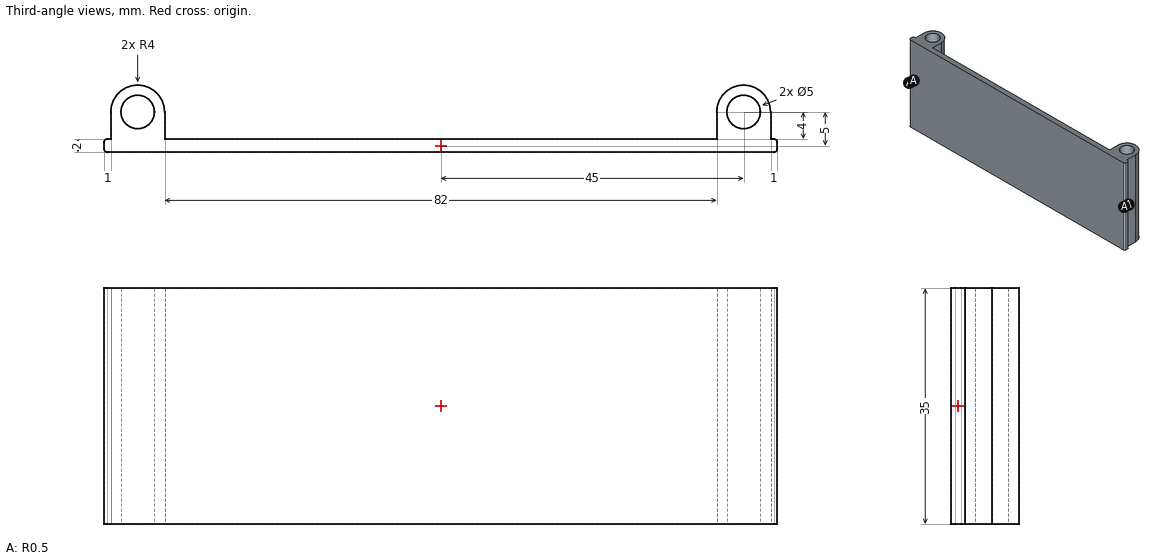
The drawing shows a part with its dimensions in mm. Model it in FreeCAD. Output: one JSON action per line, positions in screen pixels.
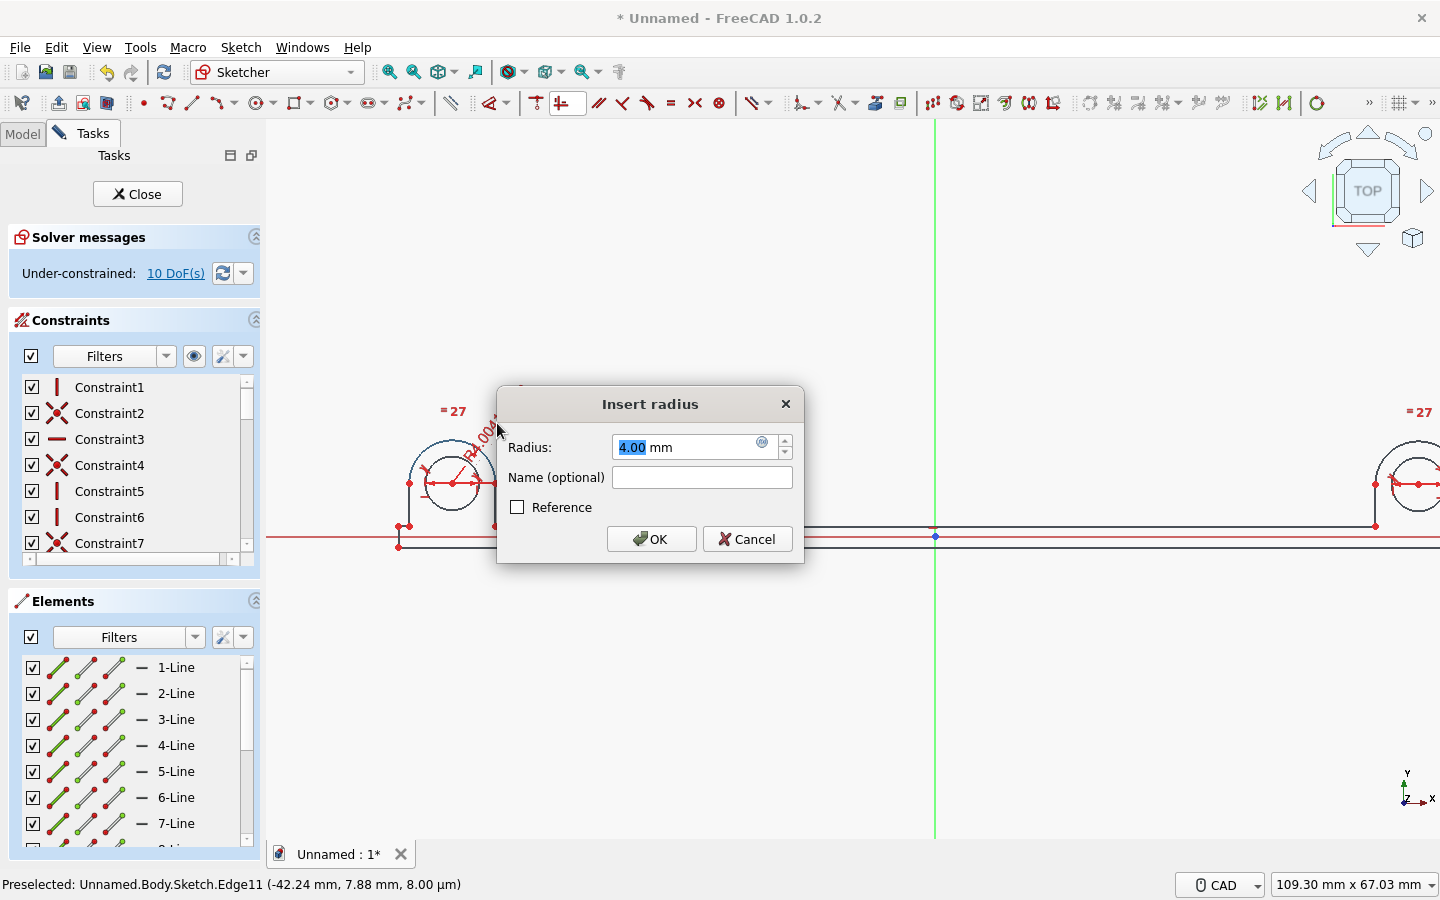
{"action": "type", "text": "4"}
{"action": "key", "text": "Return"}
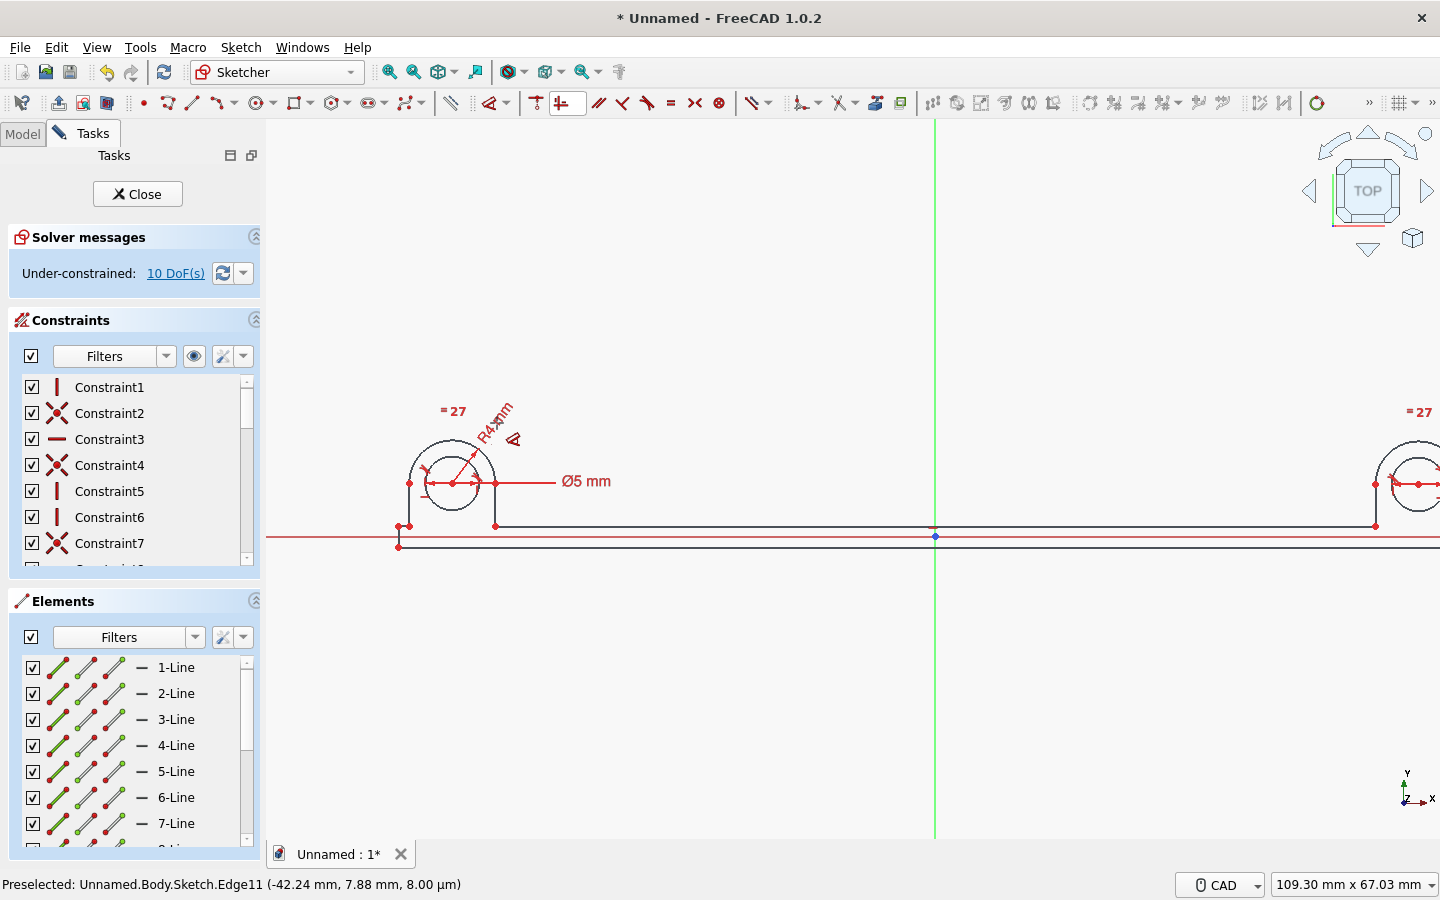
{"action": "scroll", "coordinate": [478, 449], "scroll_direction": "down", "scroll_amount": 2}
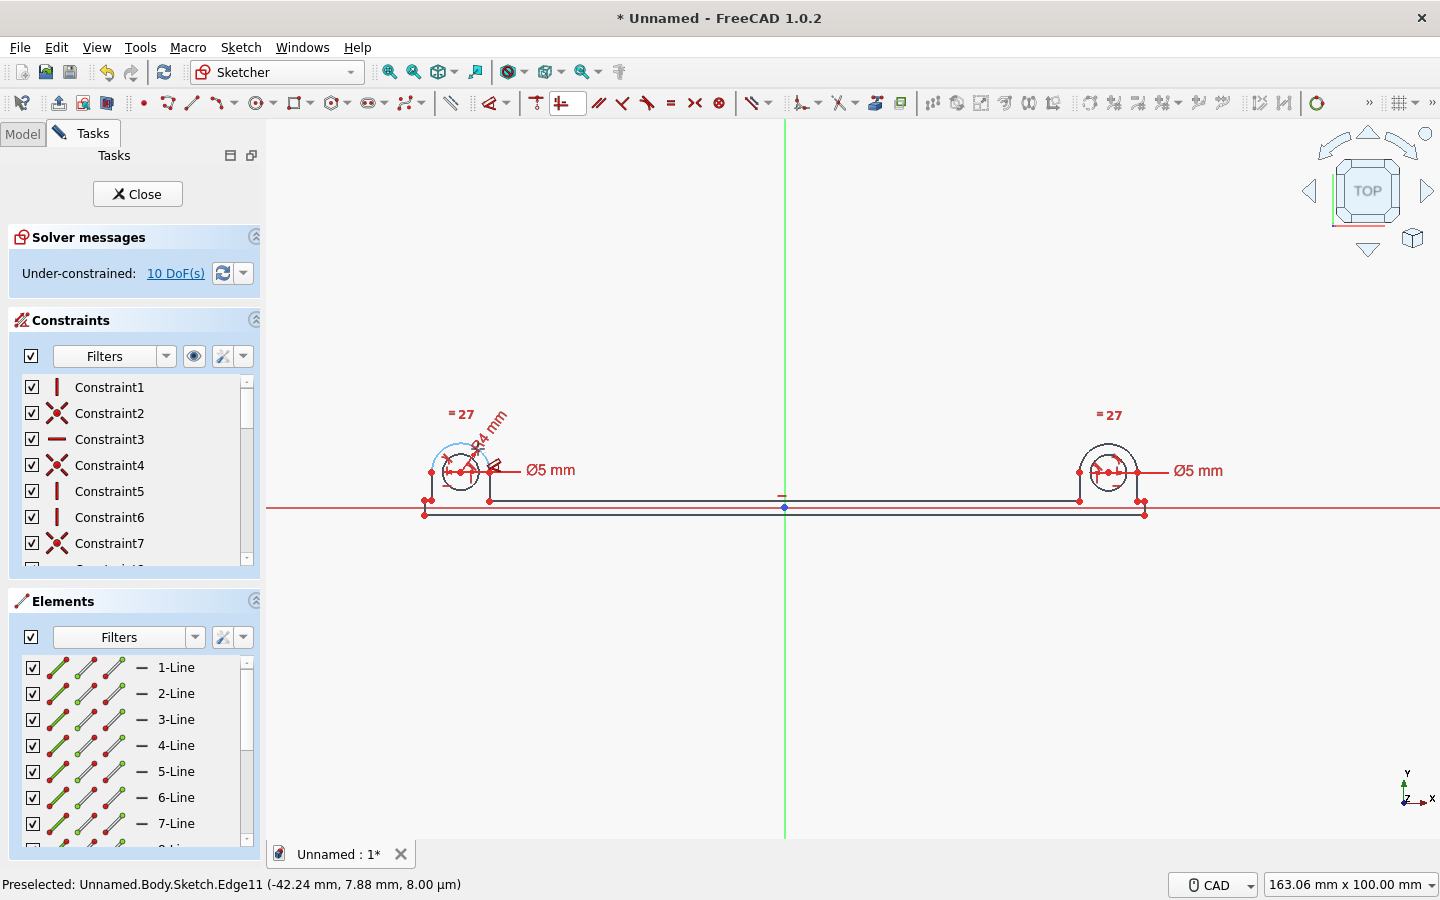
{"action": "scroll", "coordinate": [1080, 481], "scroll_direction": "up", "scroll_amount": 3}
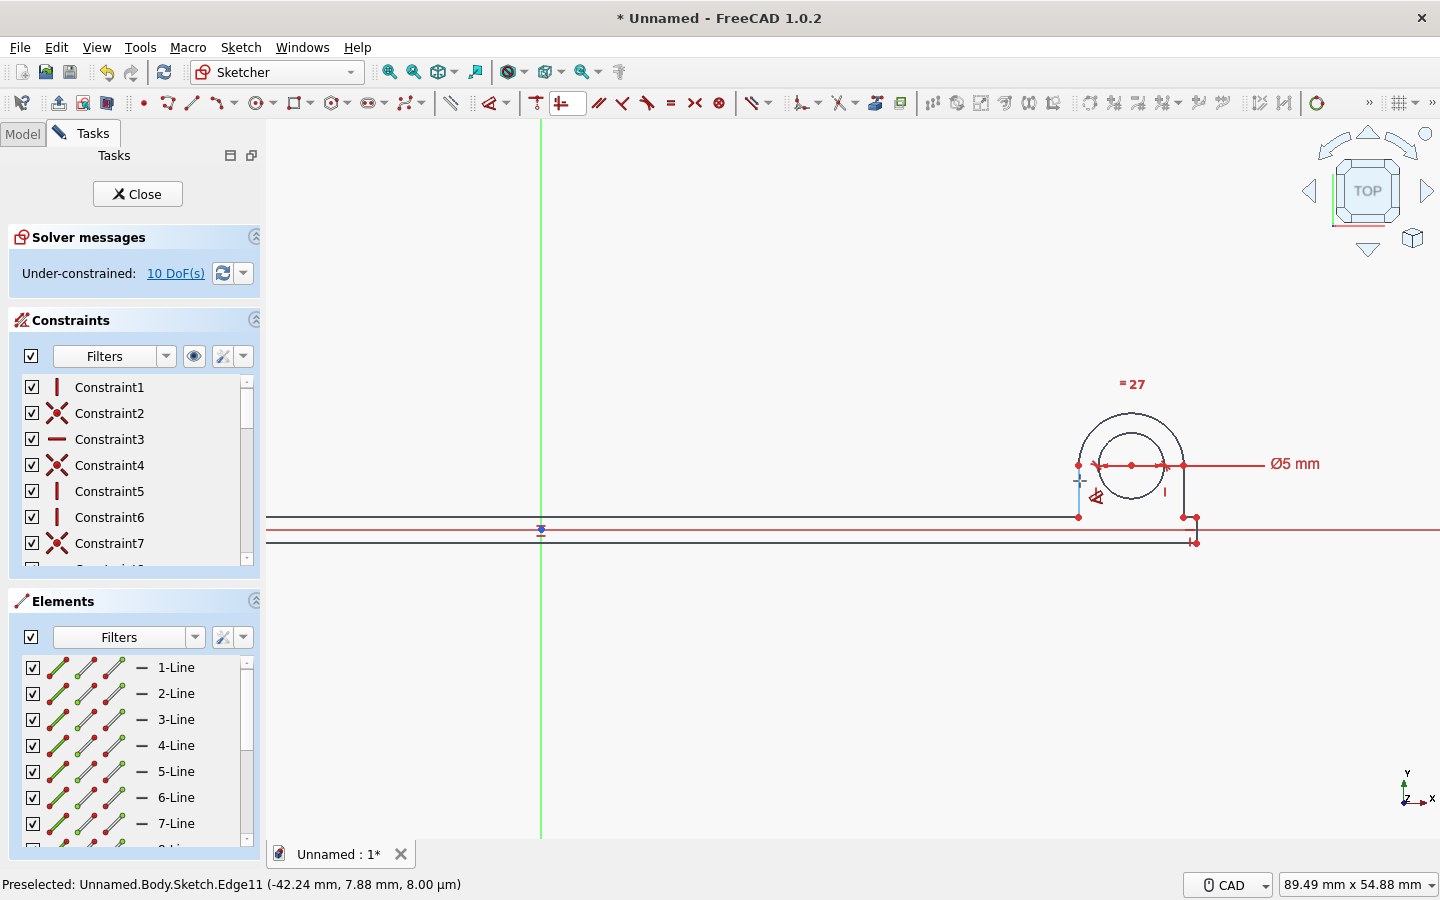
{"action": "left_click", "coordinate": [1079, 481]}
{"action": "left_click", "coordinate": [1113, 510]}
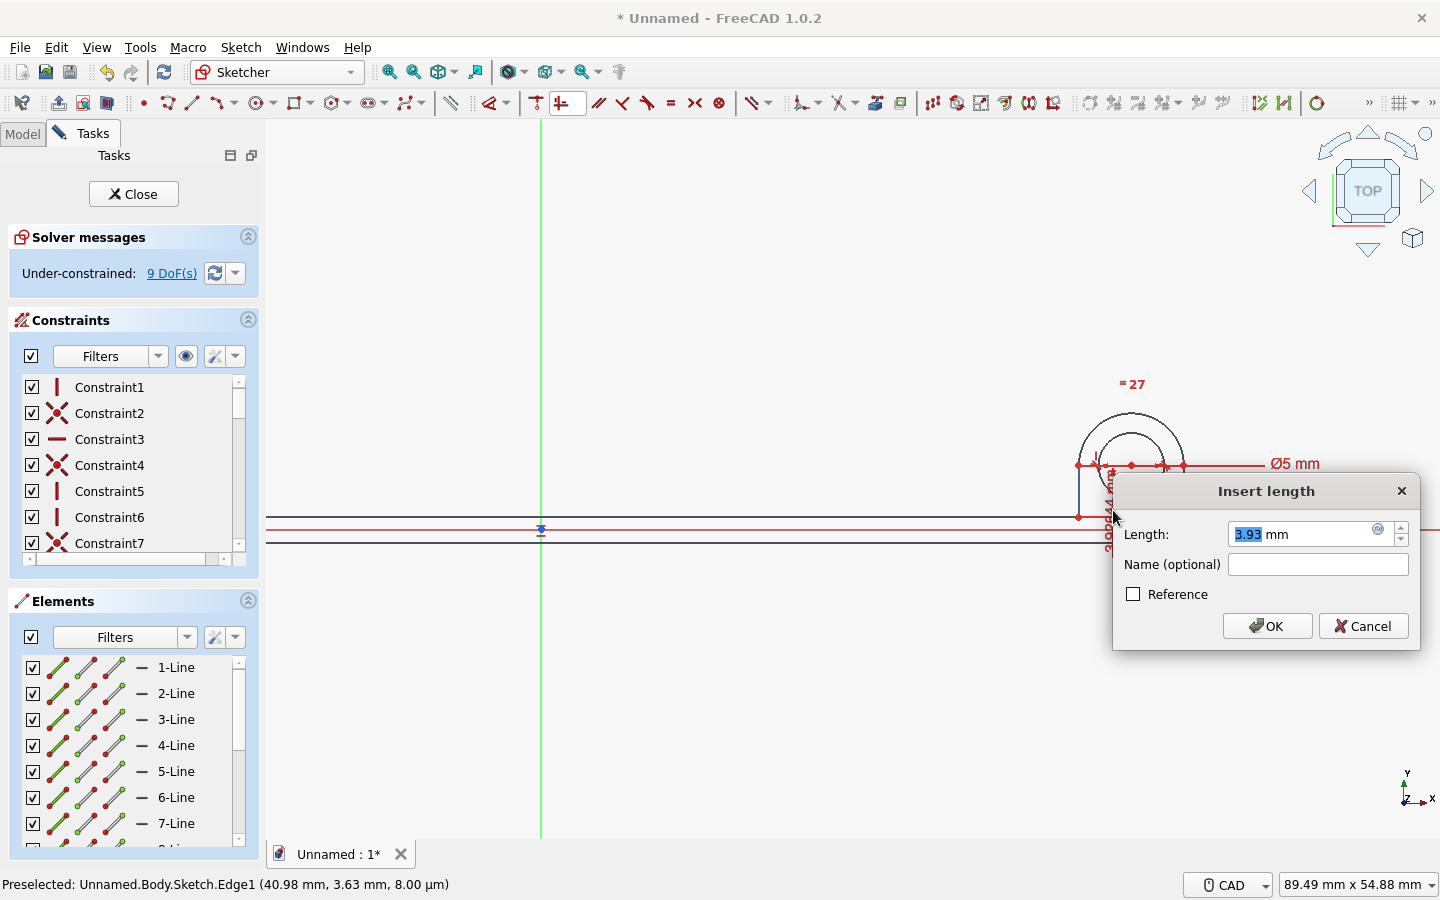
{"action": "type", "text": "4"}
{"action": "key", "text": "Return"}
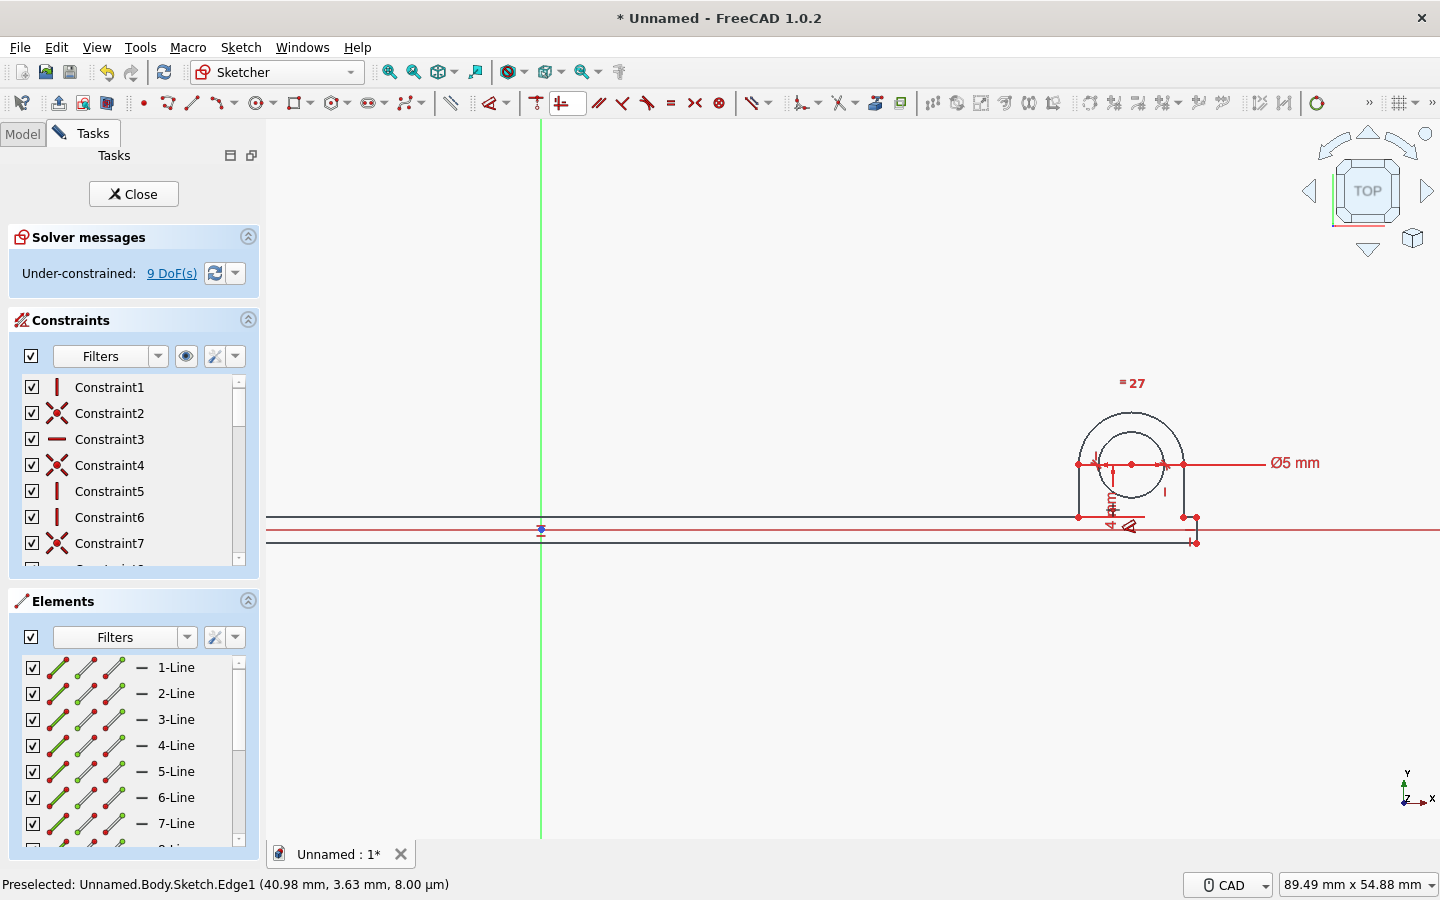
{"action": "scroll", "coordinate": [1080, 481], "scroll_direction": "down", "scroll_amount": 3}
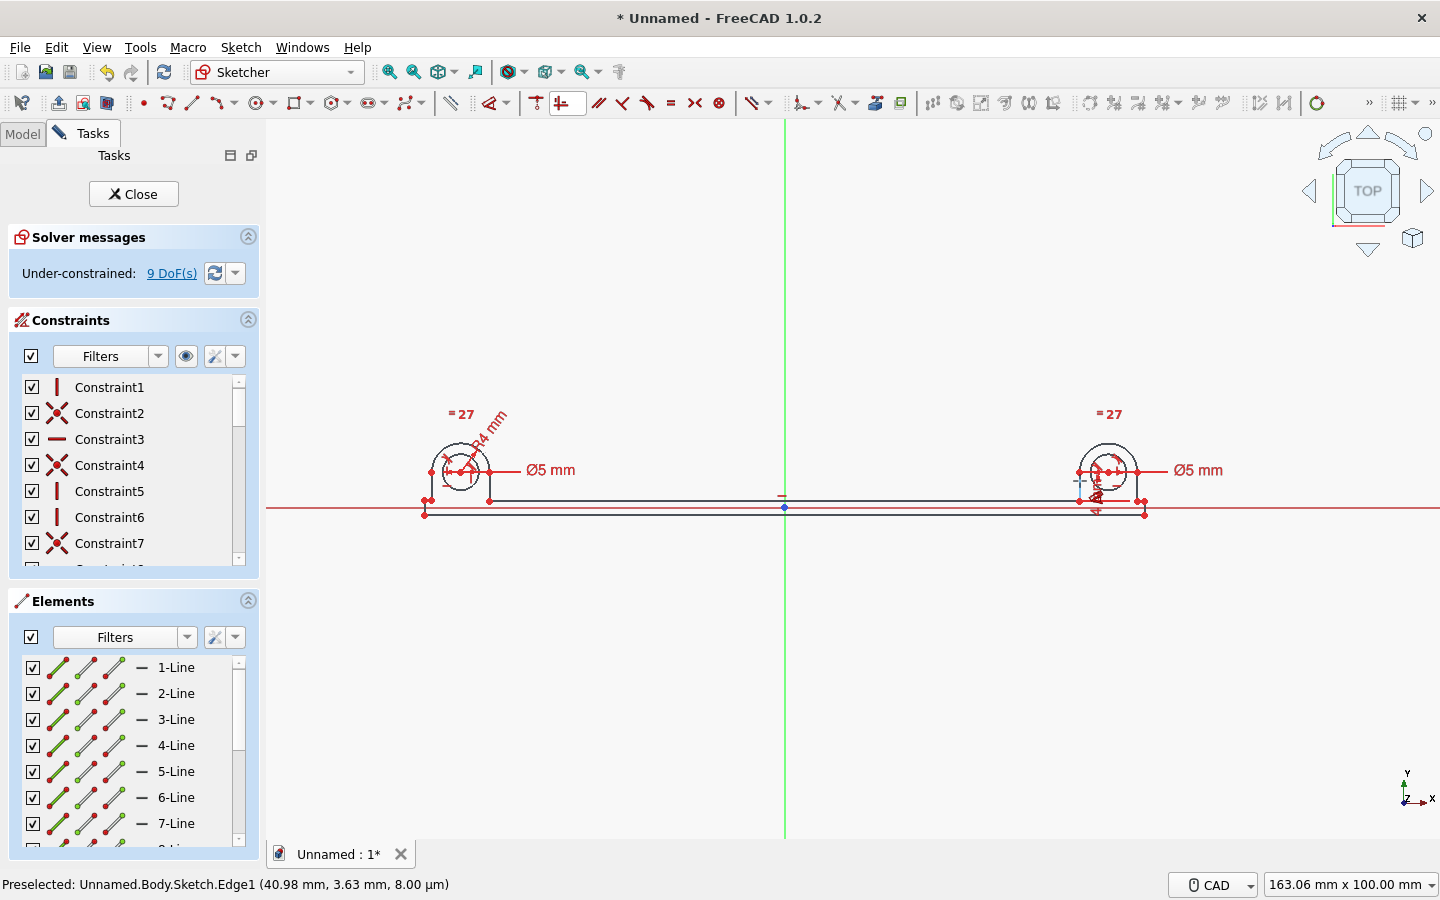
{"action": "scroll", "coordinate": [490, 493], "scroll_direction": "up", "scroll_amount": 3}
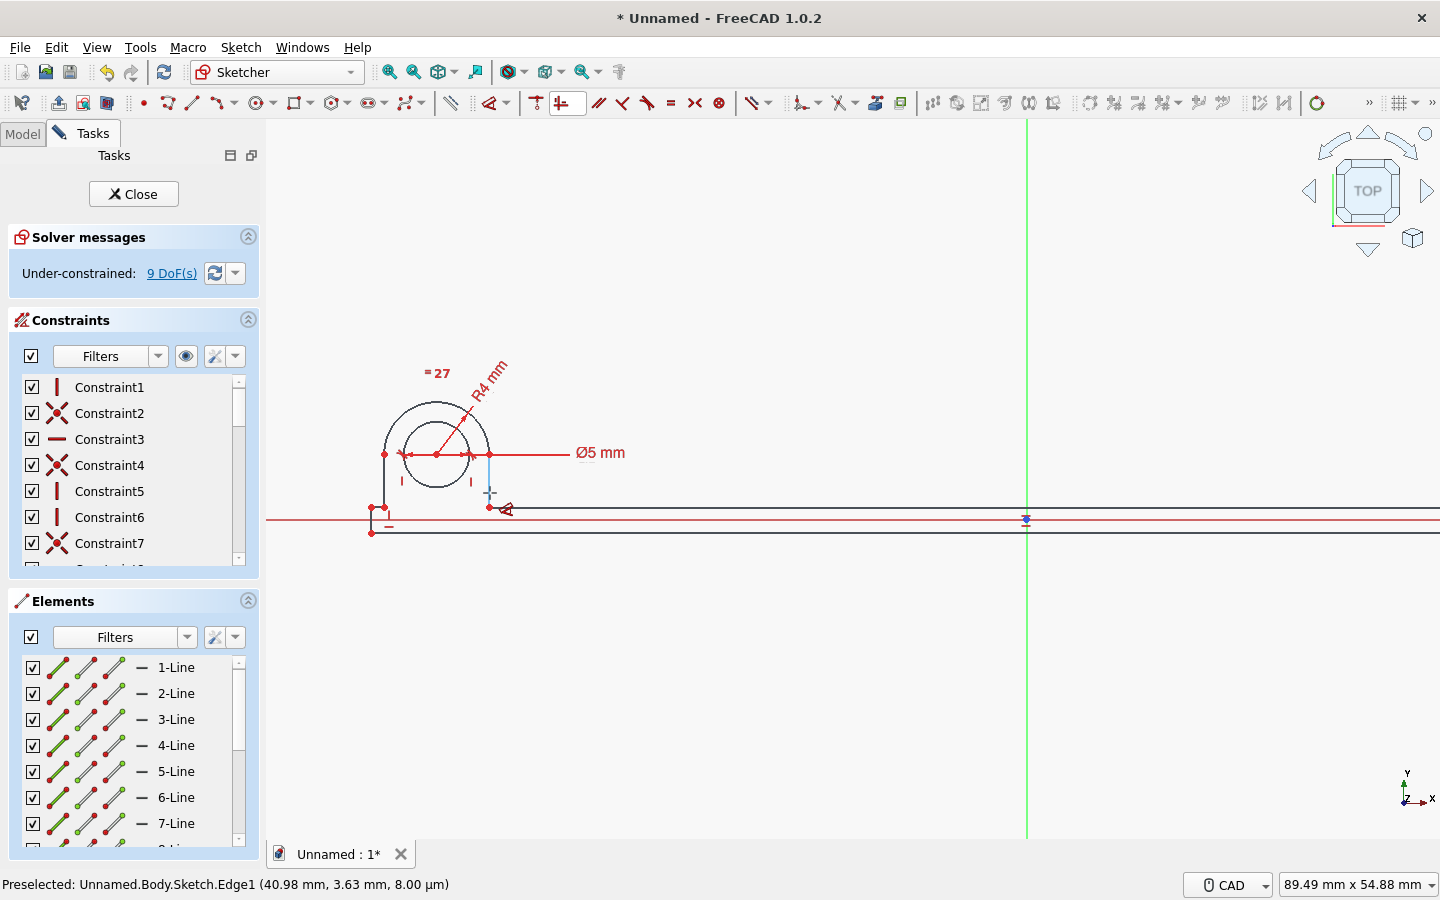
{"action": "left_click", "coordinate": [489, 492]}
{"action": "left_click", "coordinate": [455, 500]}